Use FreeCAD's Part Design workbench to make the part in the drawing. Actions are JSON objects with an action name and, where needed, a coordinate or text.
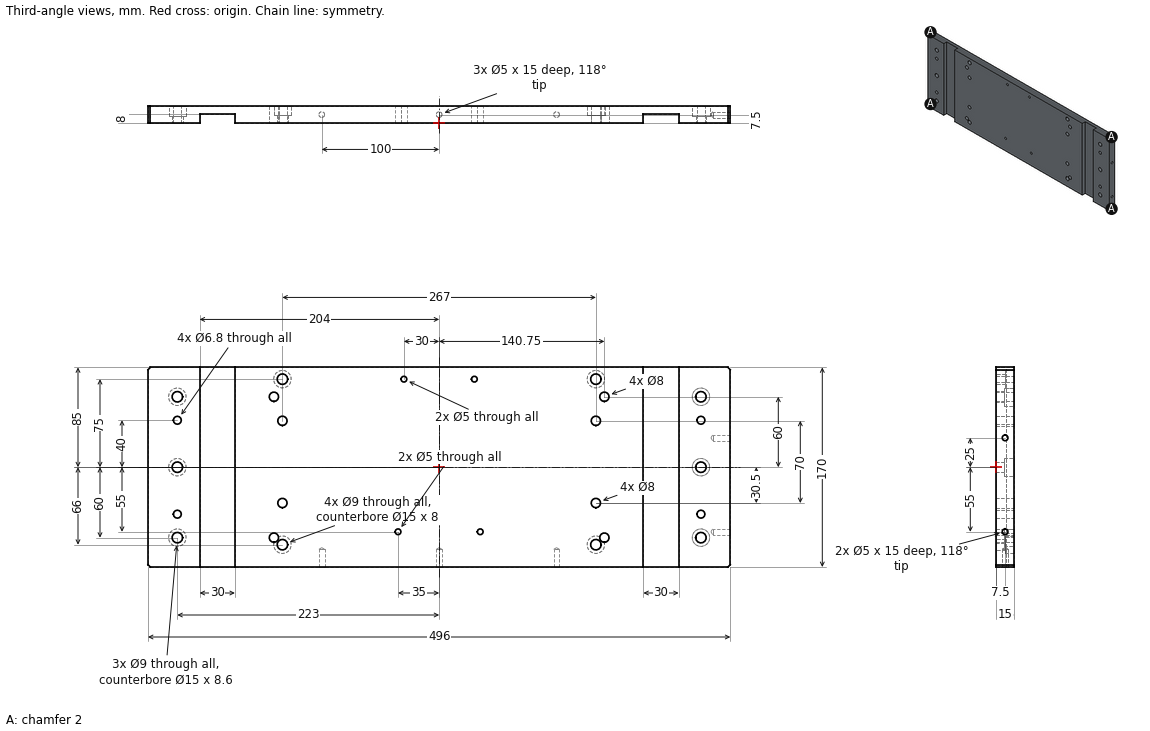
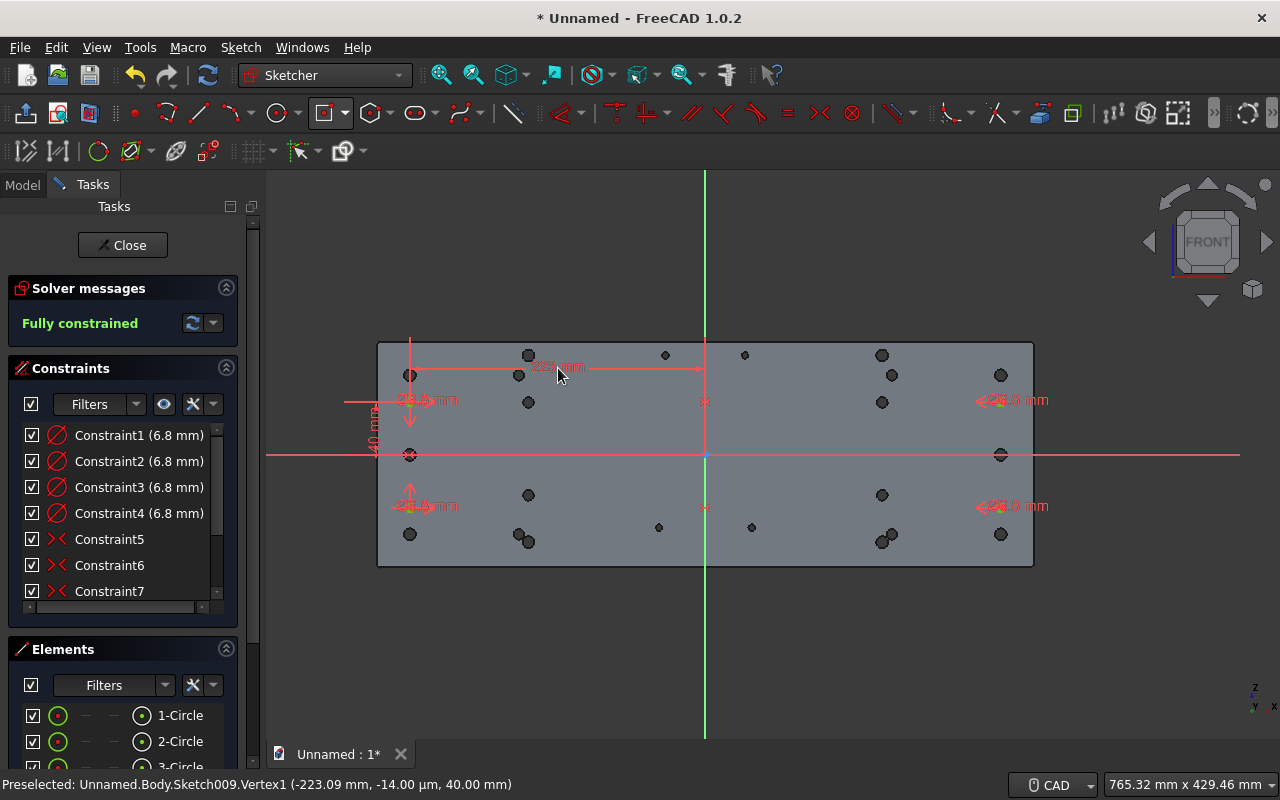
{"action": "left_click", "coordinate": [123, 245]}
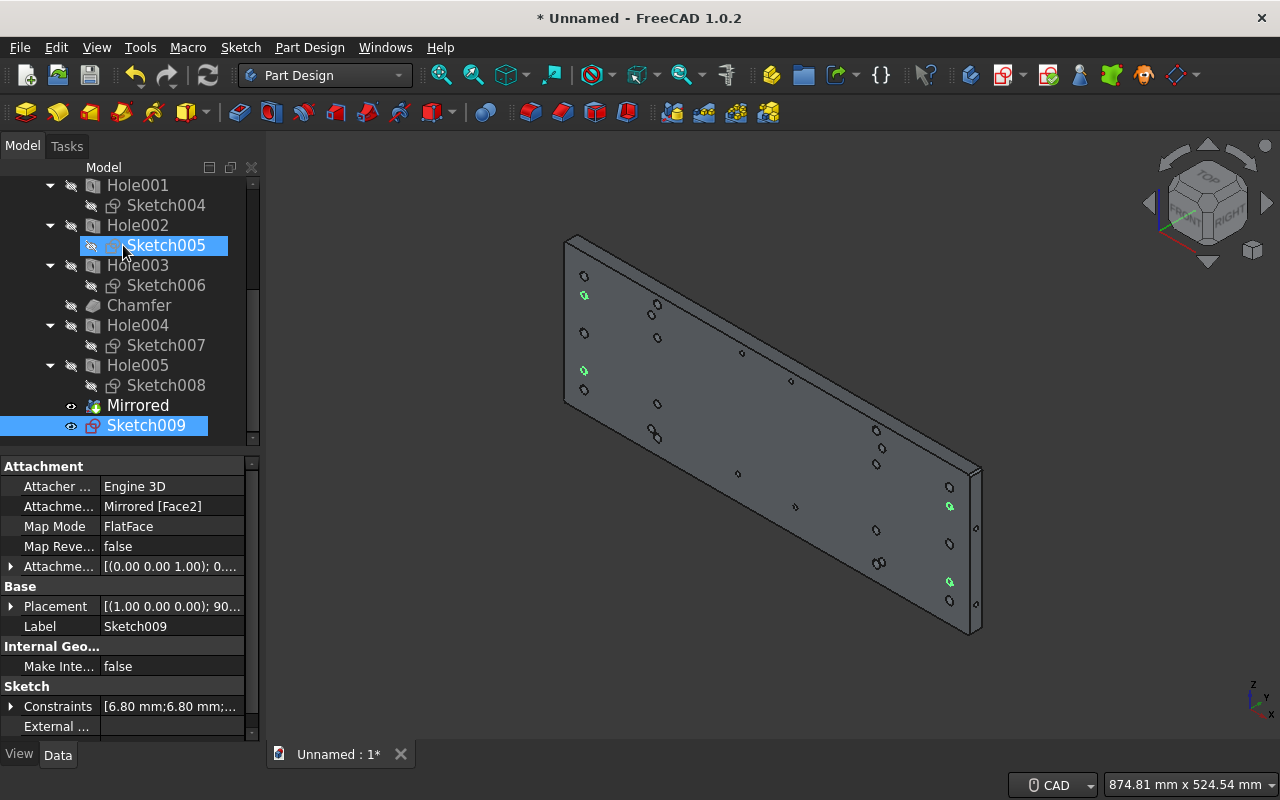
{"action": "left_click", "coordinate": [272, 112]}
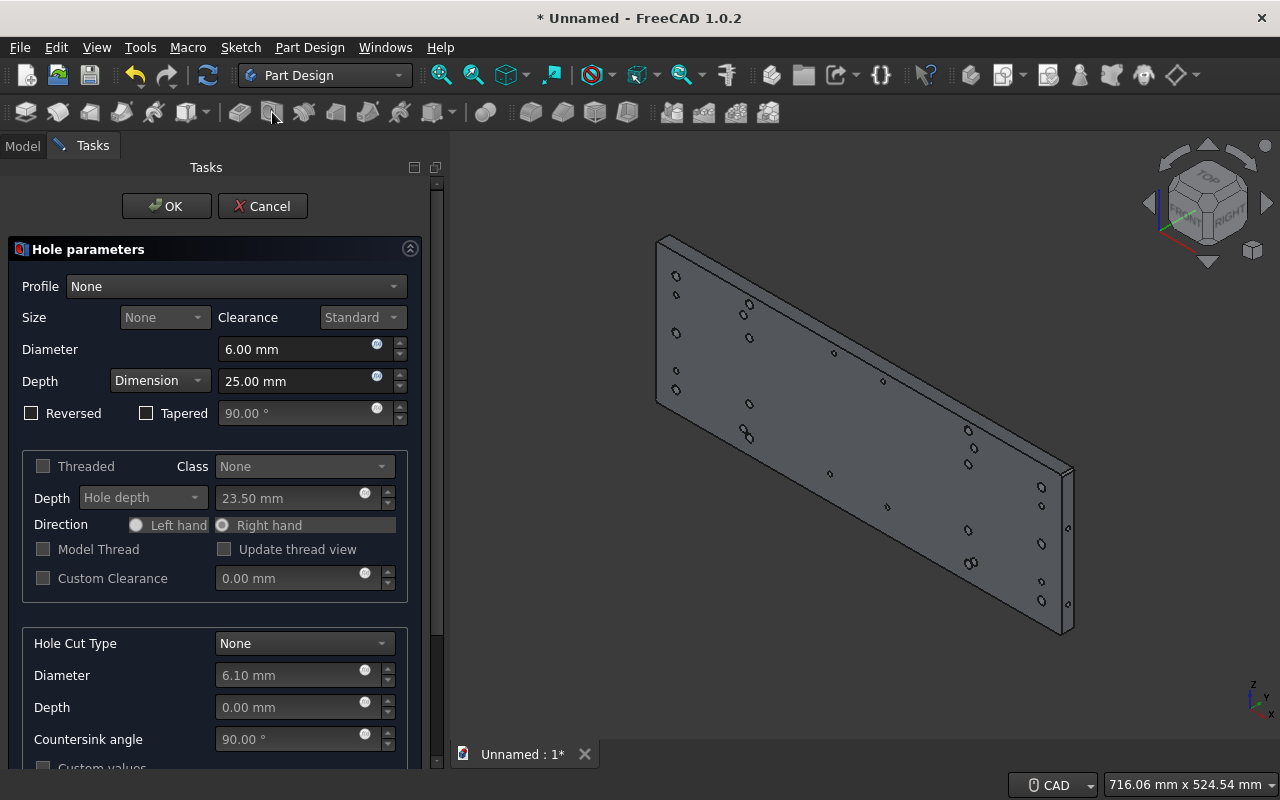
{"action": "triple_click", "coordinate": [305, 349]}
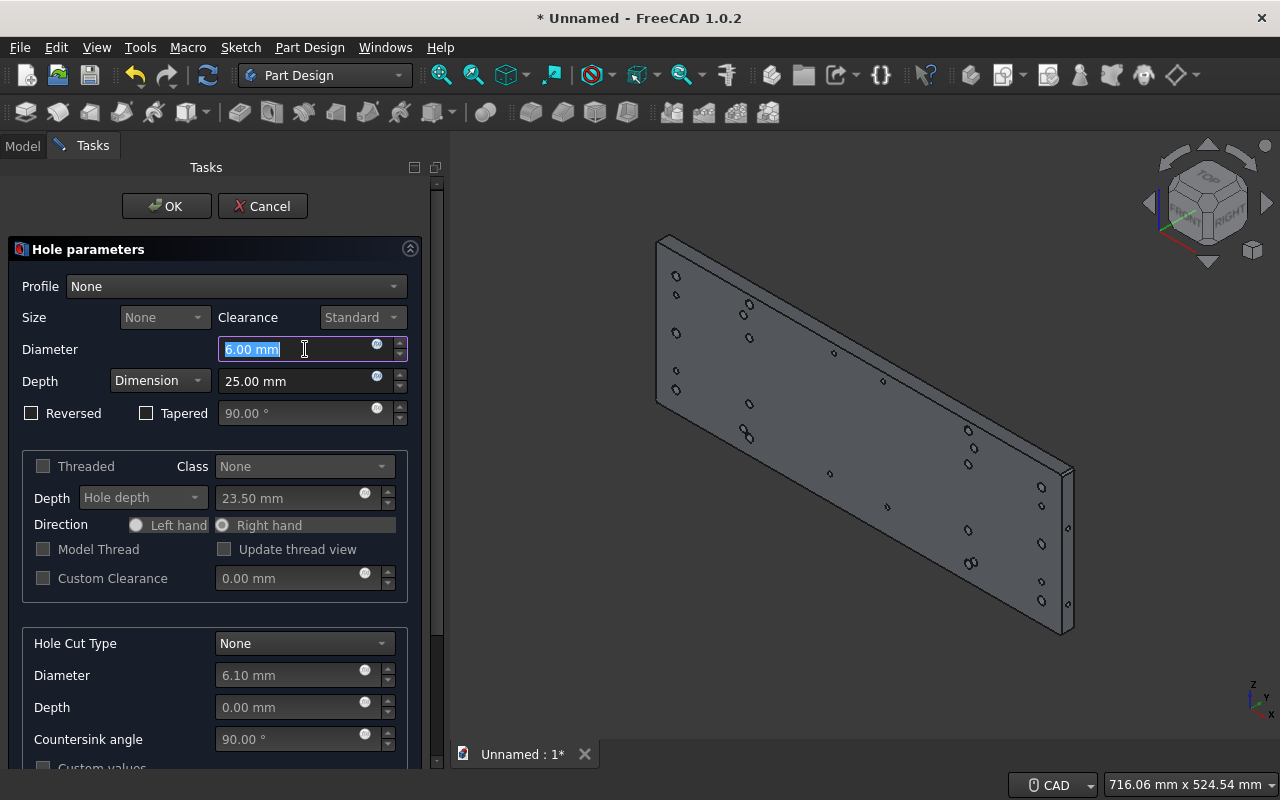
{"action": "type", "text": "6.8"}
{"action": "key", "text": "Tab"}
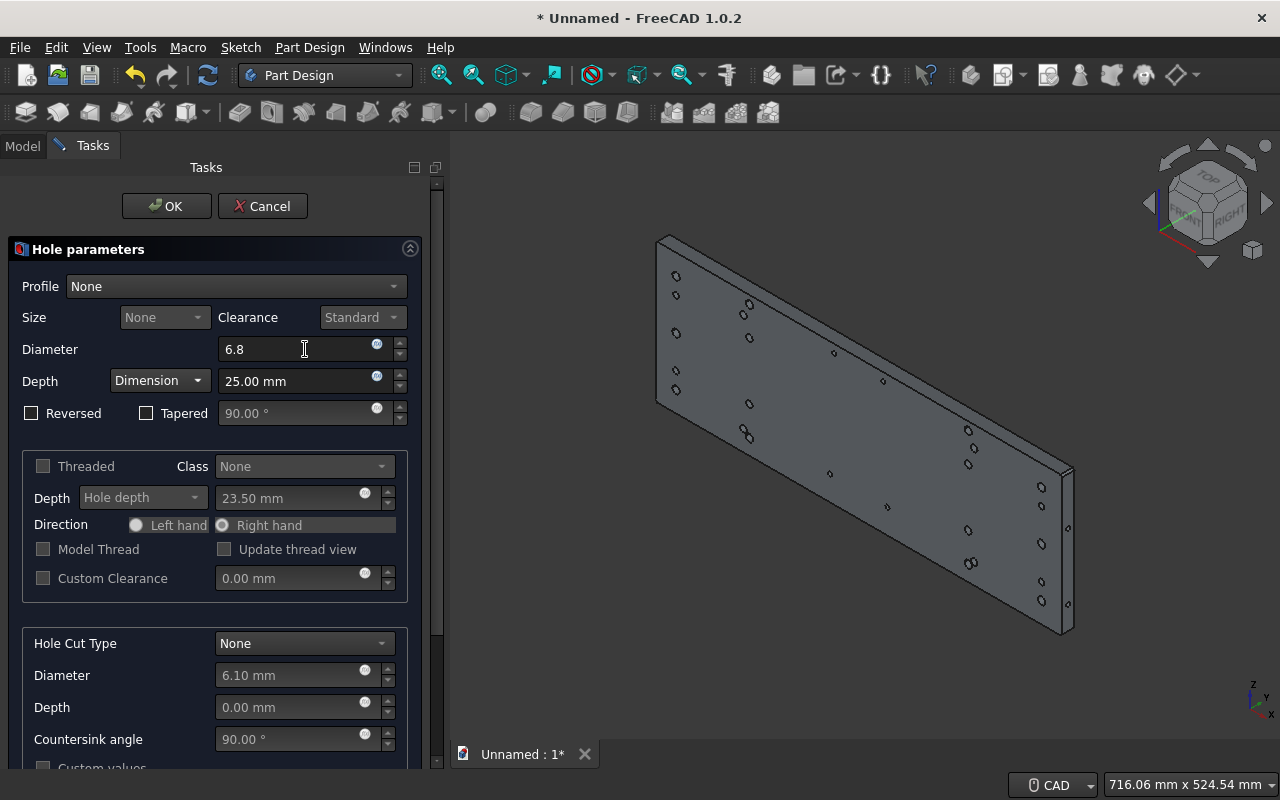
{"action": "left_click", "coordinate": [161, 380]}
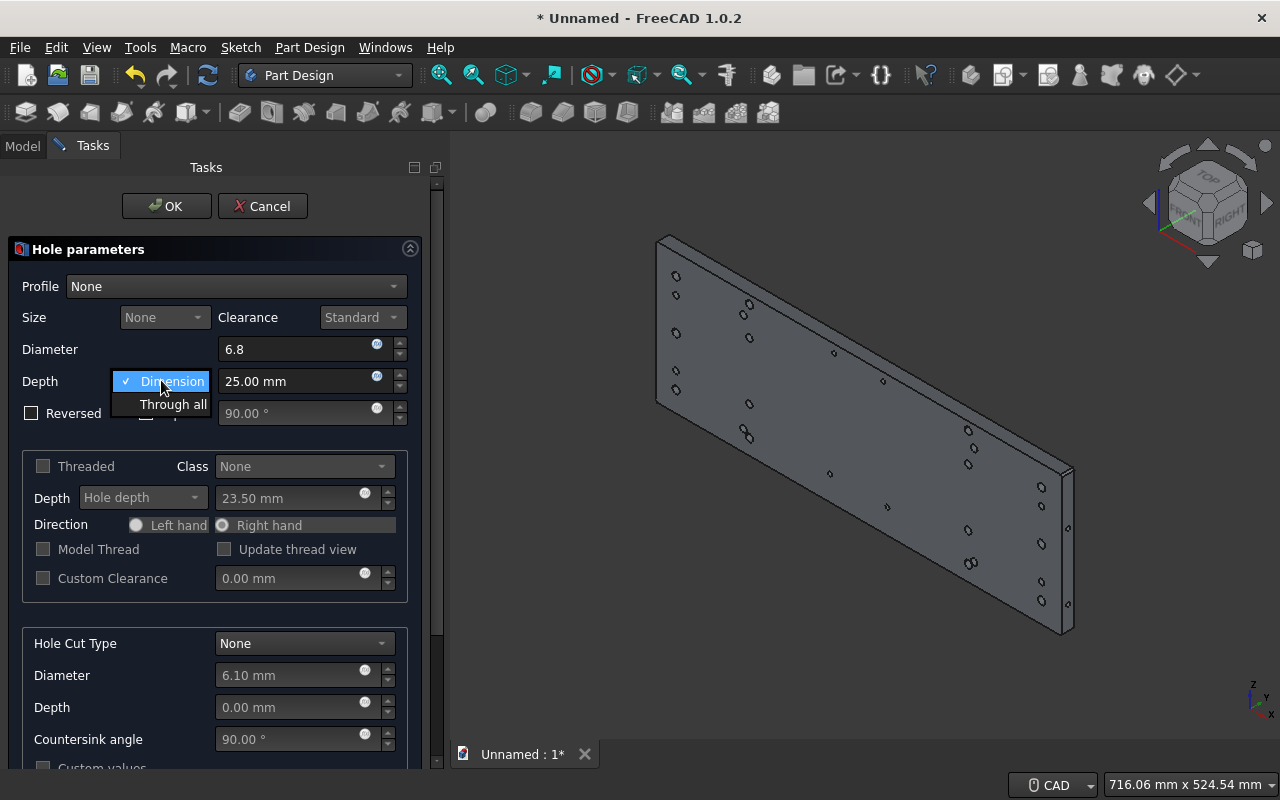
{"action": "left_click", "coordinate": [160, 404]}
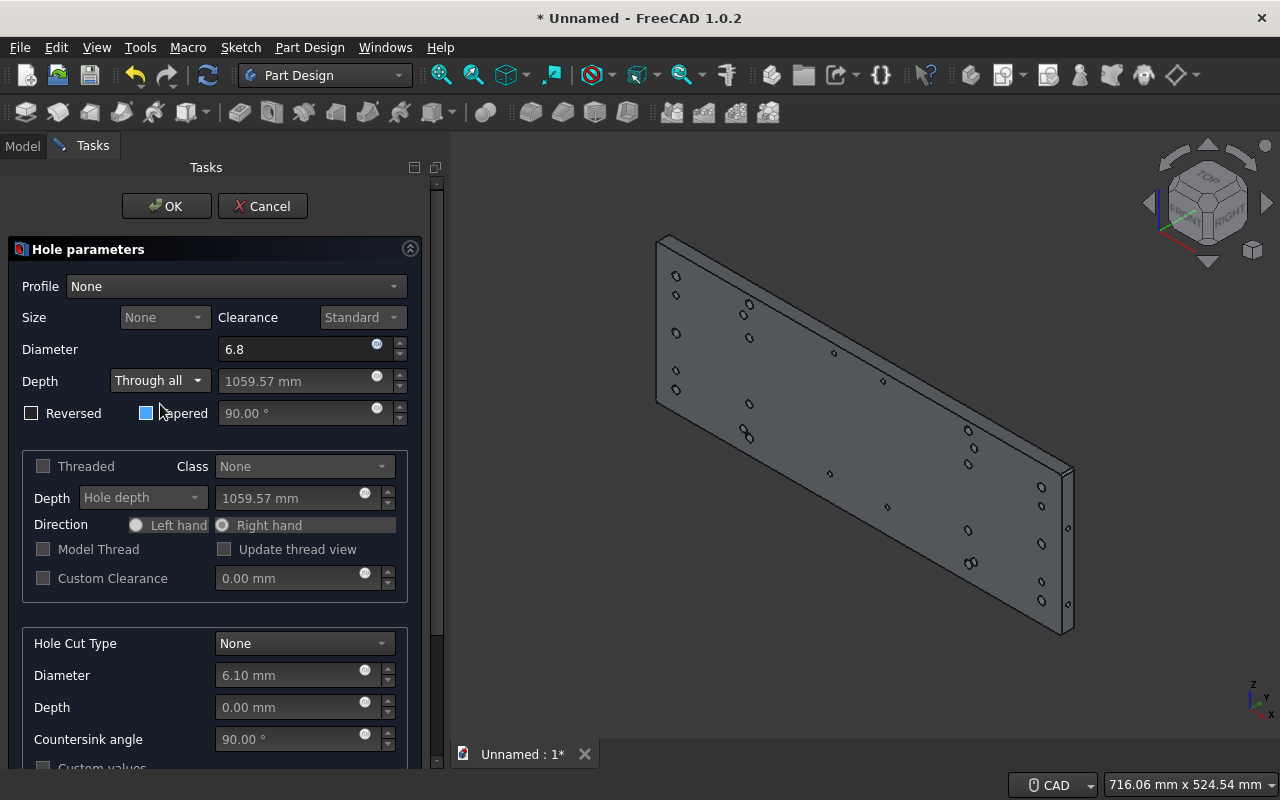
{"action": "left_click", "coordinate": [167, 206]}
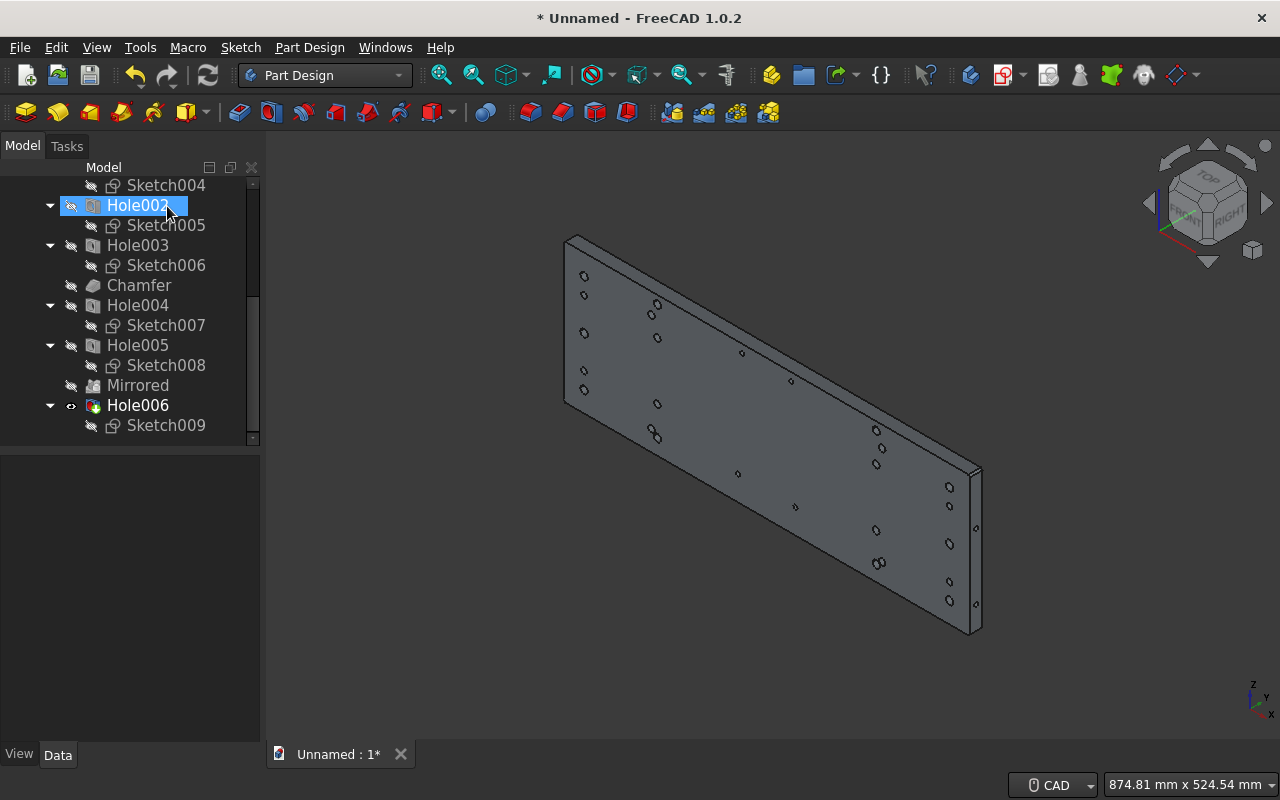
{"action": "left_click", "coordinate": [1004, 76]}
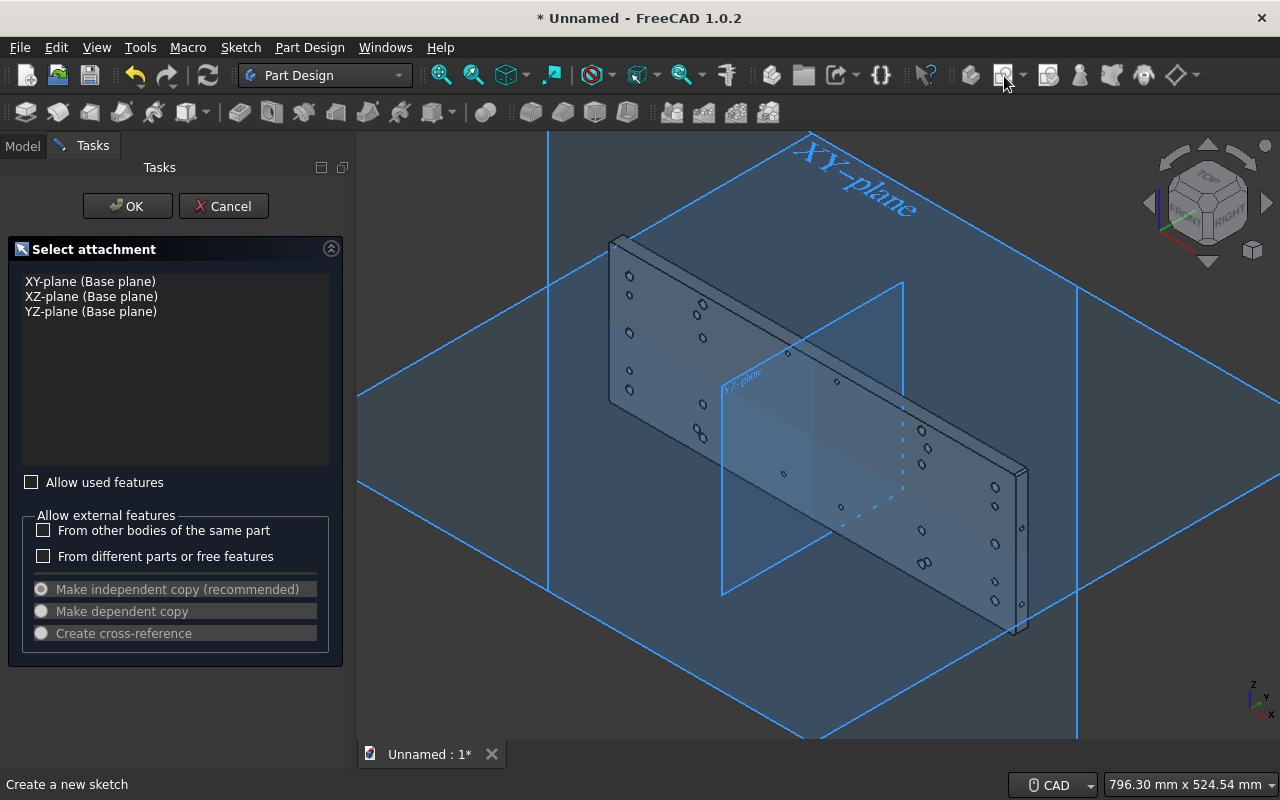
{"action": "left_click", "coordinate": [82, 296]}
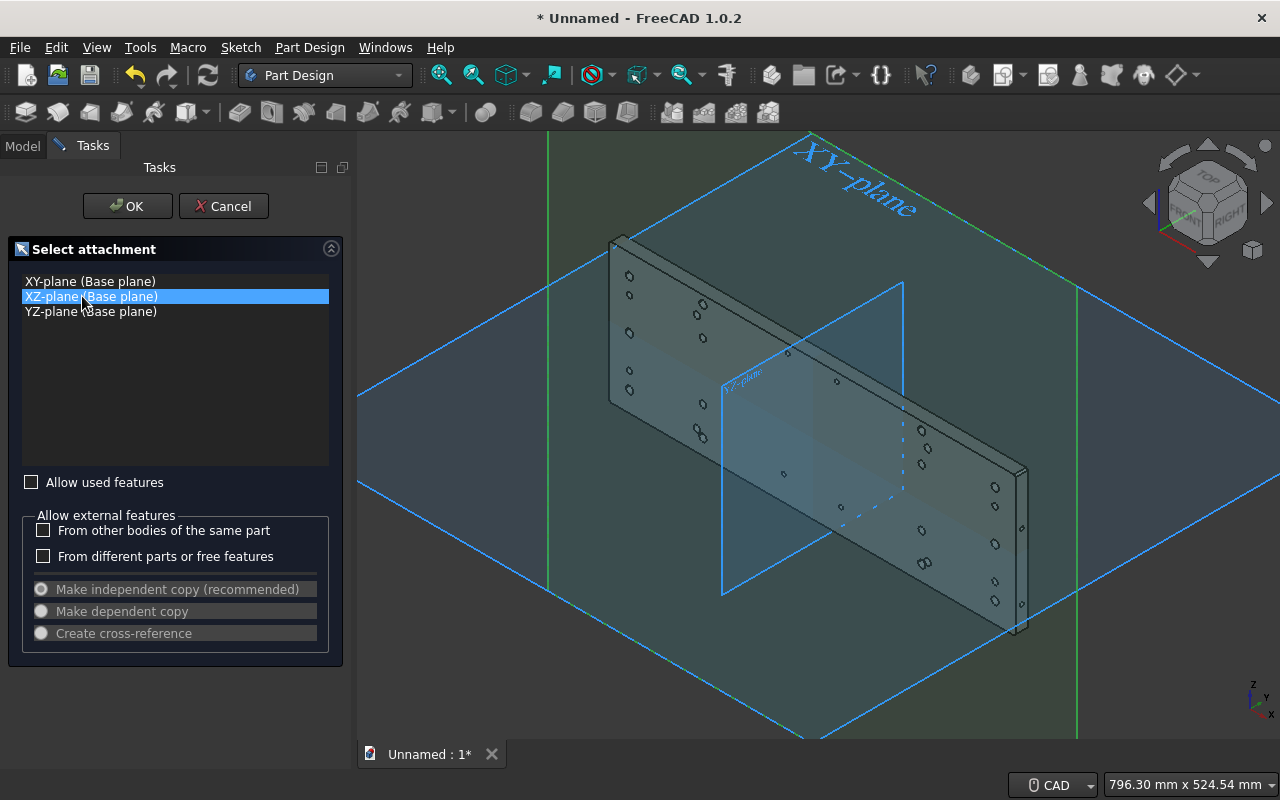
{"action": "left_click", "coordinate": [128, 206]}